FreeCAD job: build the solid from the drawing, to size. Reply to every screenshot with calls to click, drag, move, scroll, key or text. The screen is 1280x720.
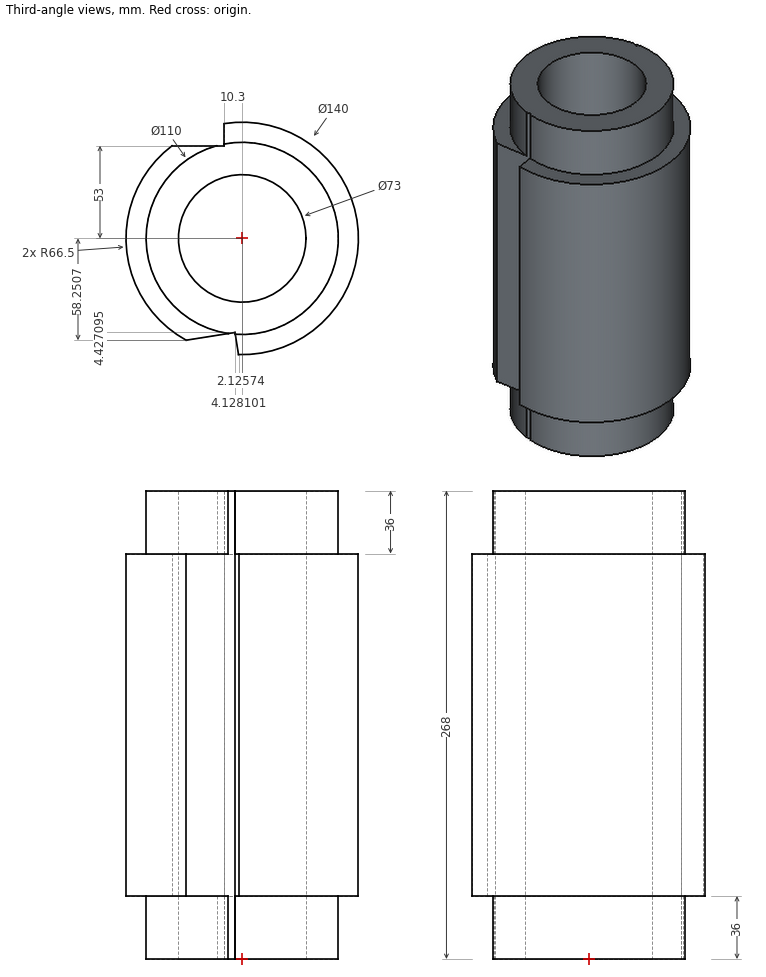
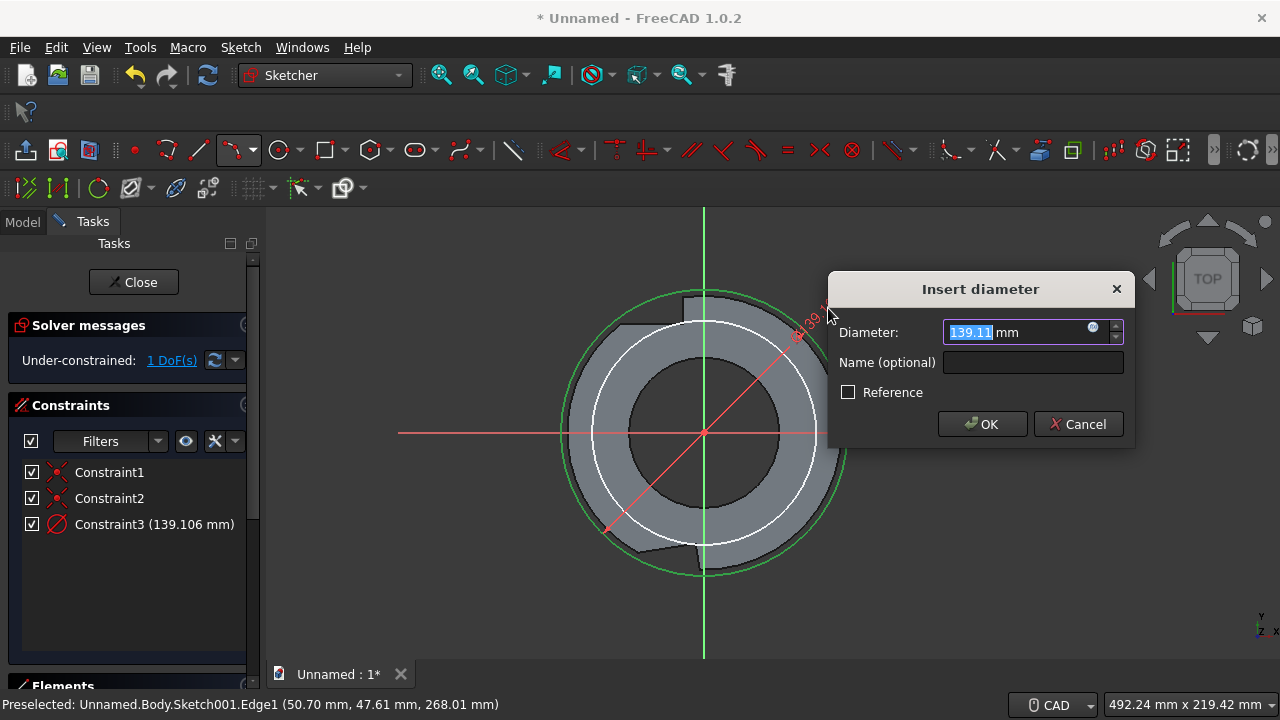
text(140)
key(Return)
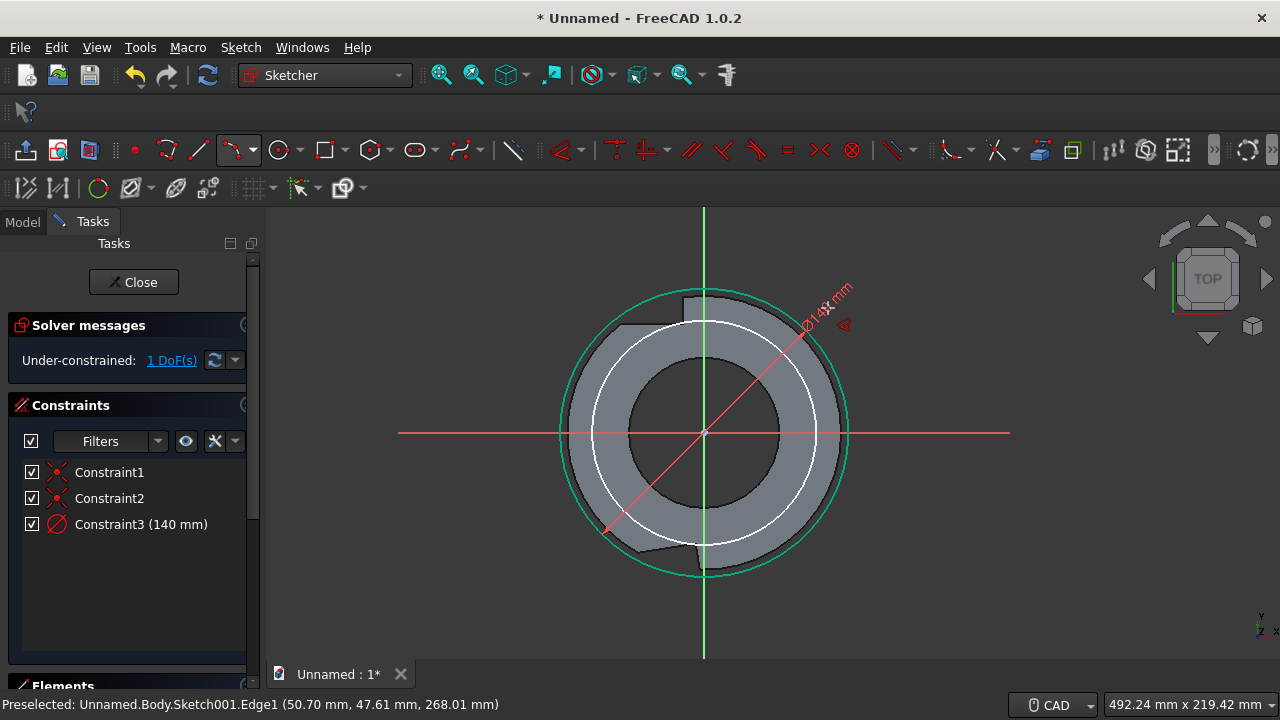
click(783, 353)
click(864, 385)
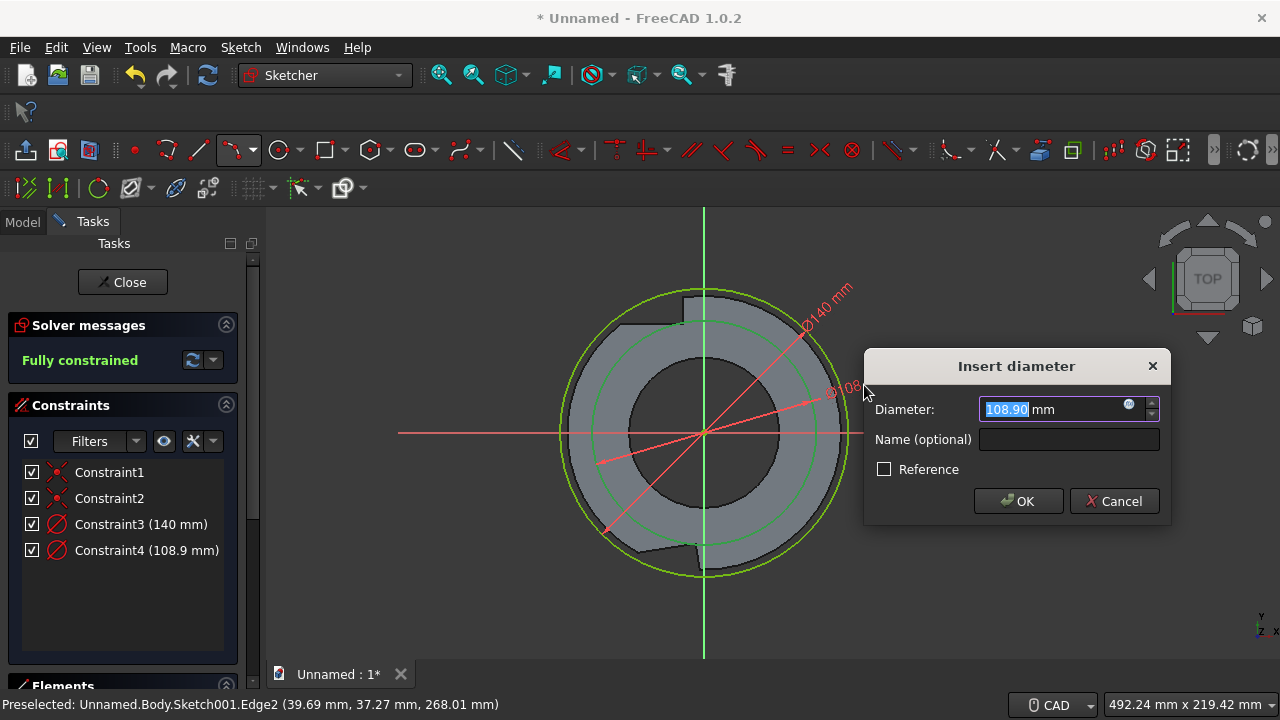
text(110)
key(Return)
key(Escape)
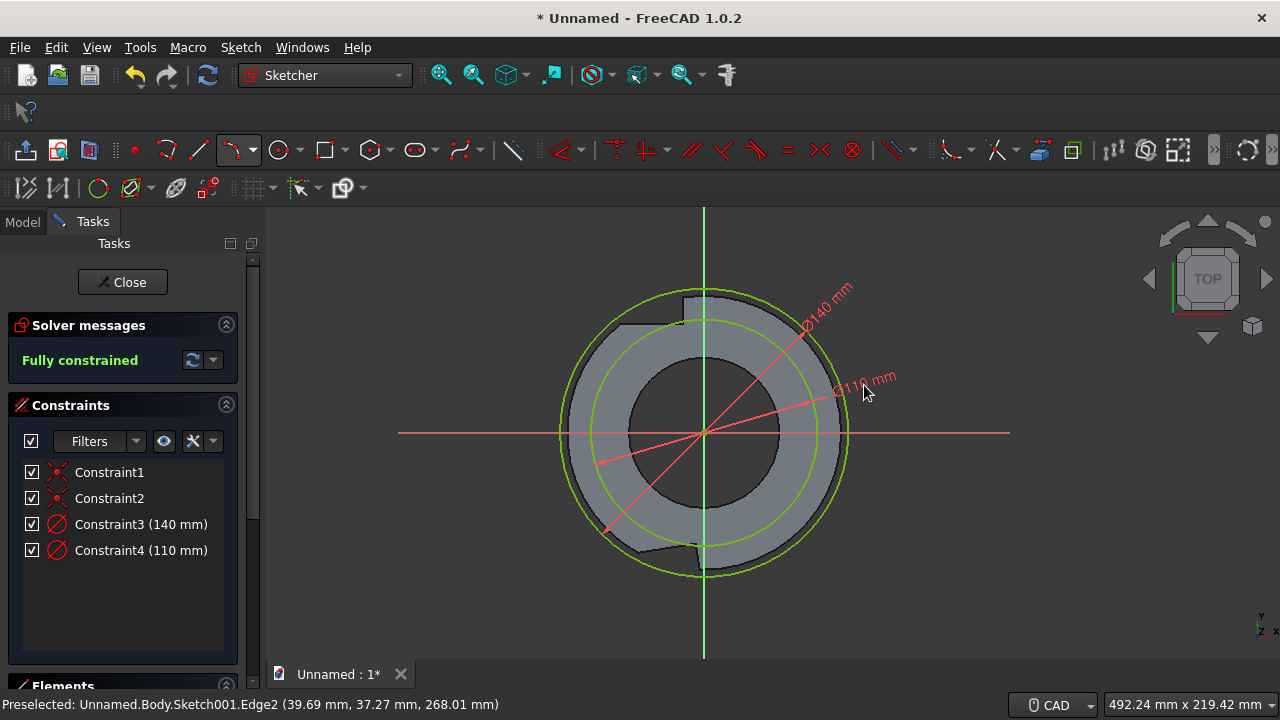
click(123, 282)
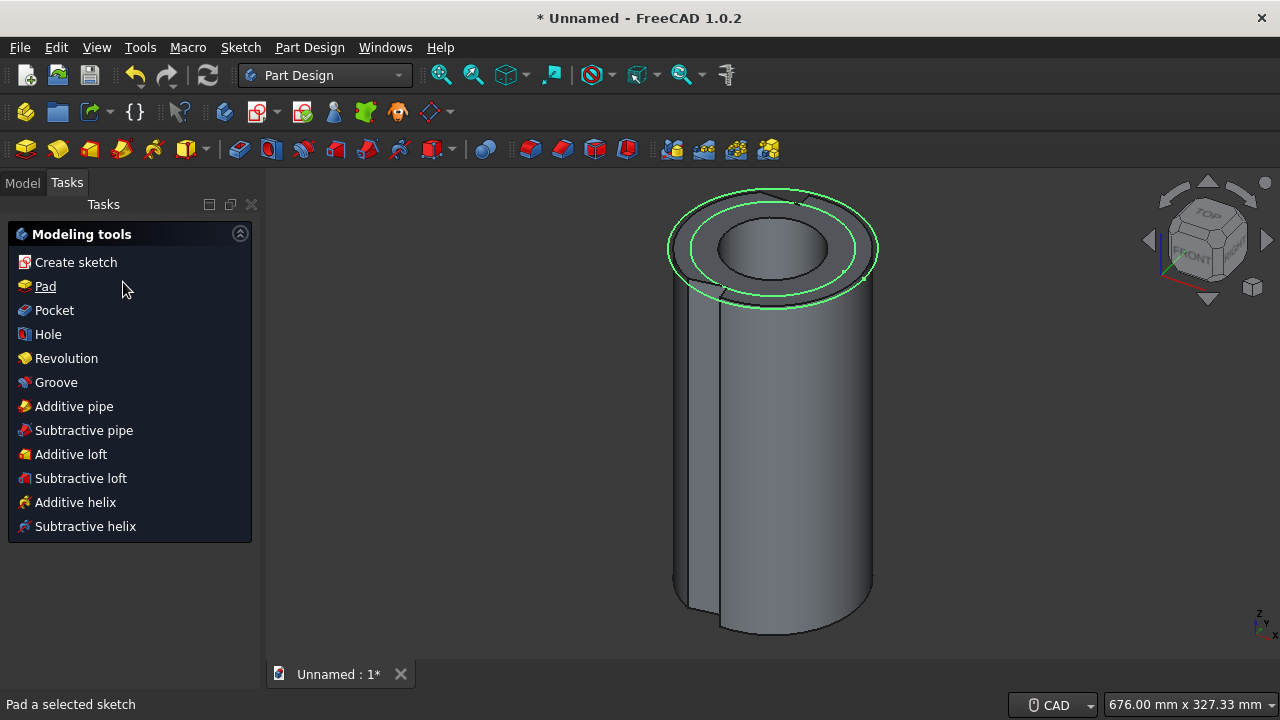
click(240, 150)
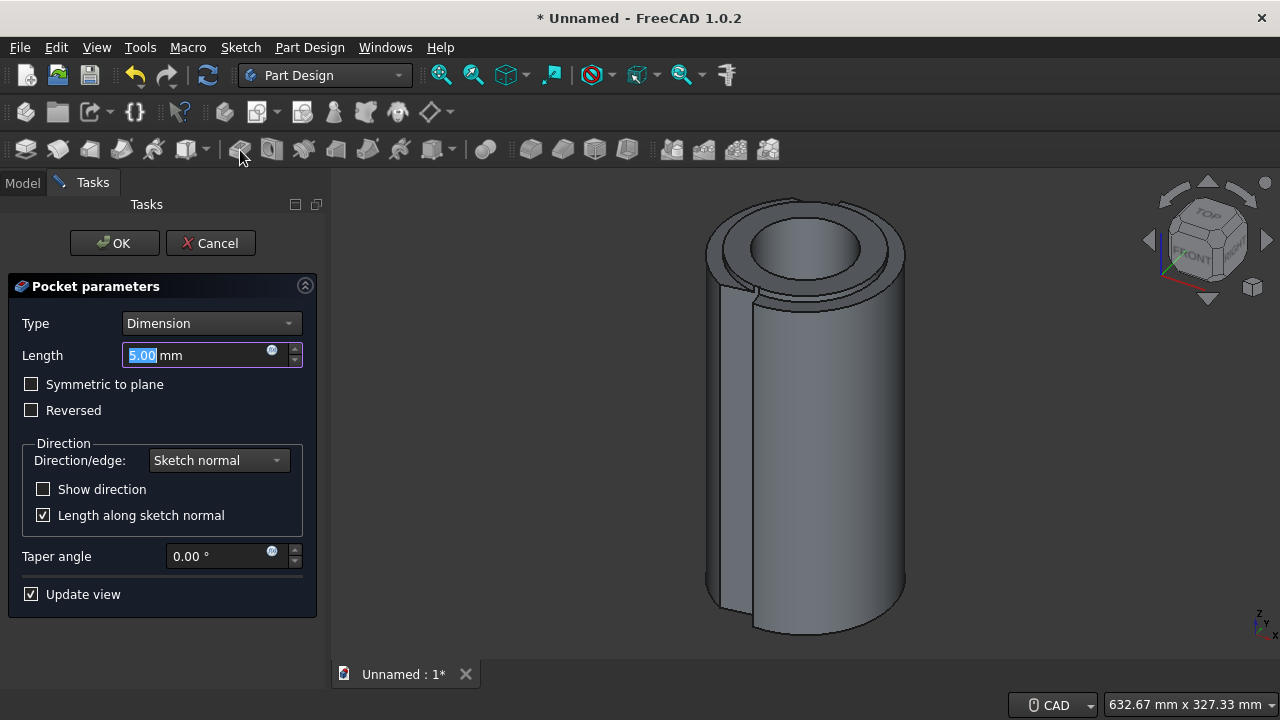
text(36)
key(Tab)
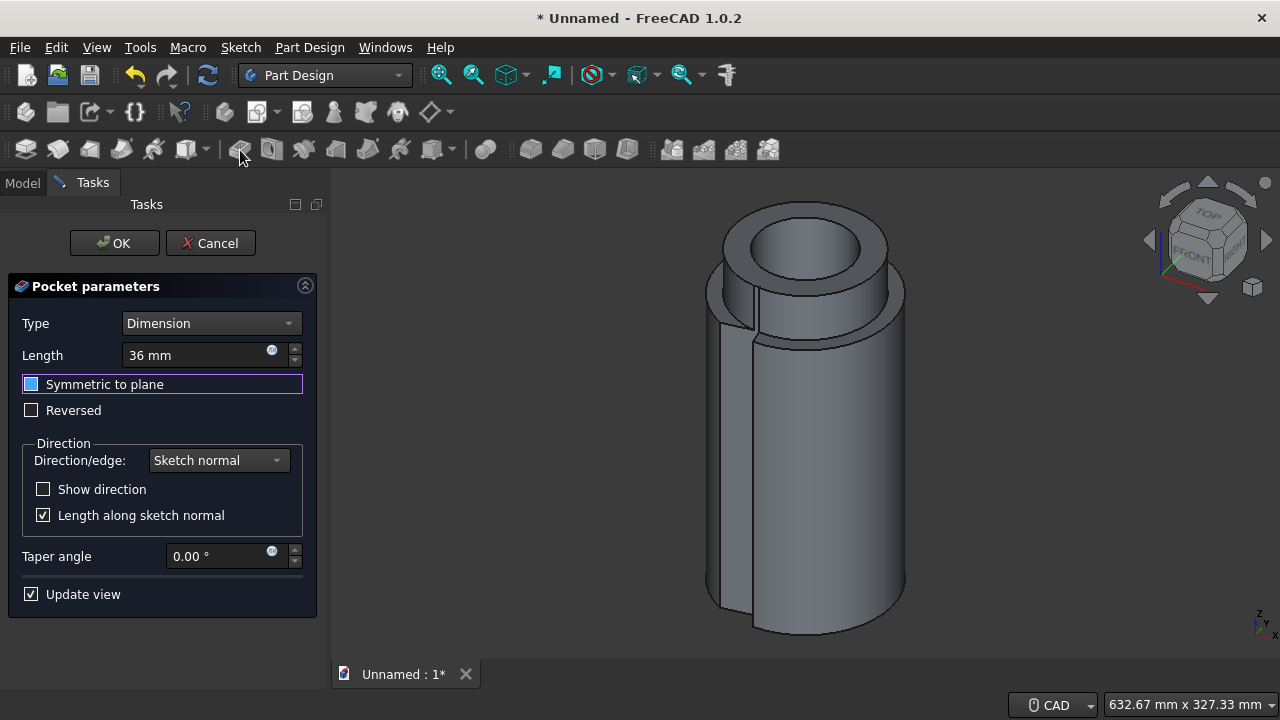
click(115, 243)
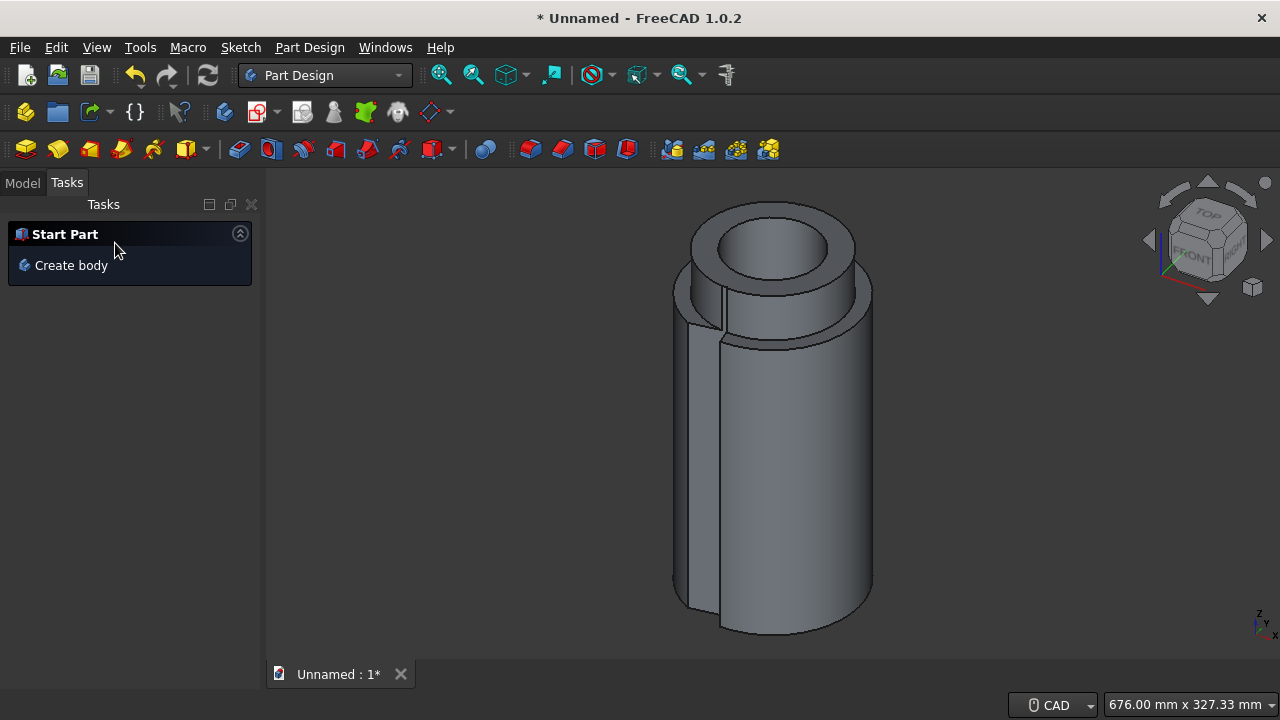
click(23, 182)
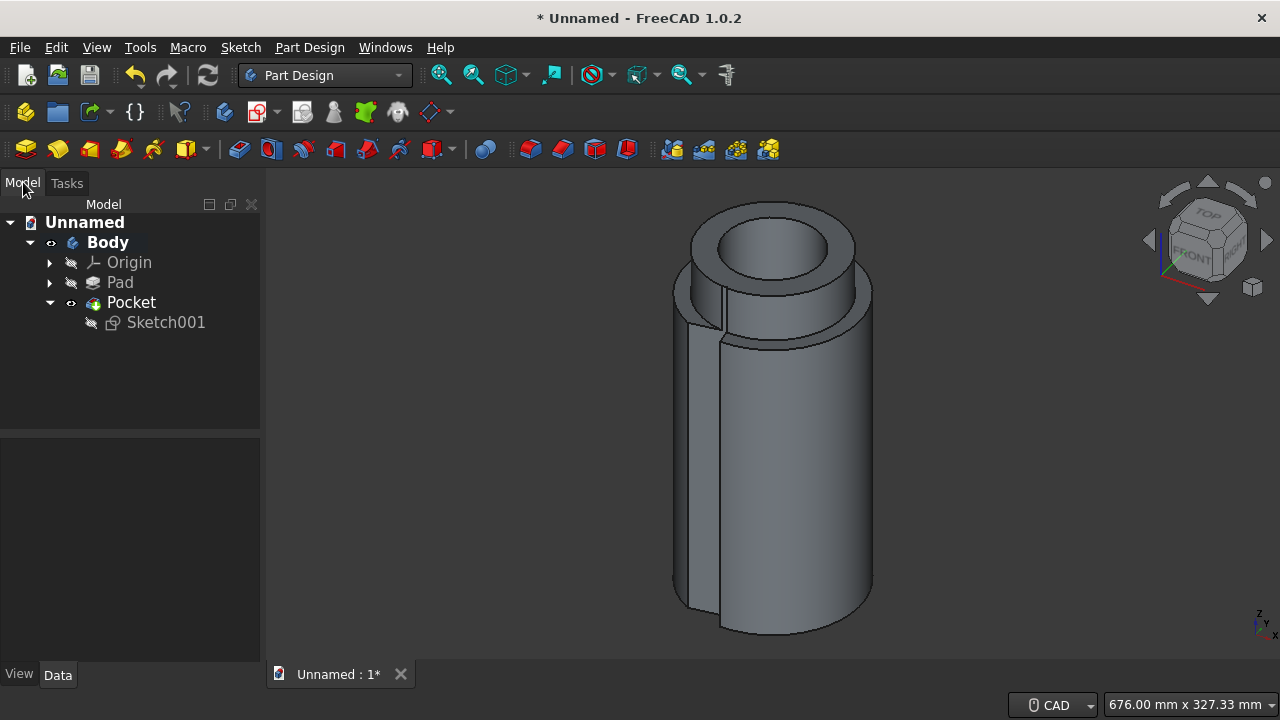
click(50, 263)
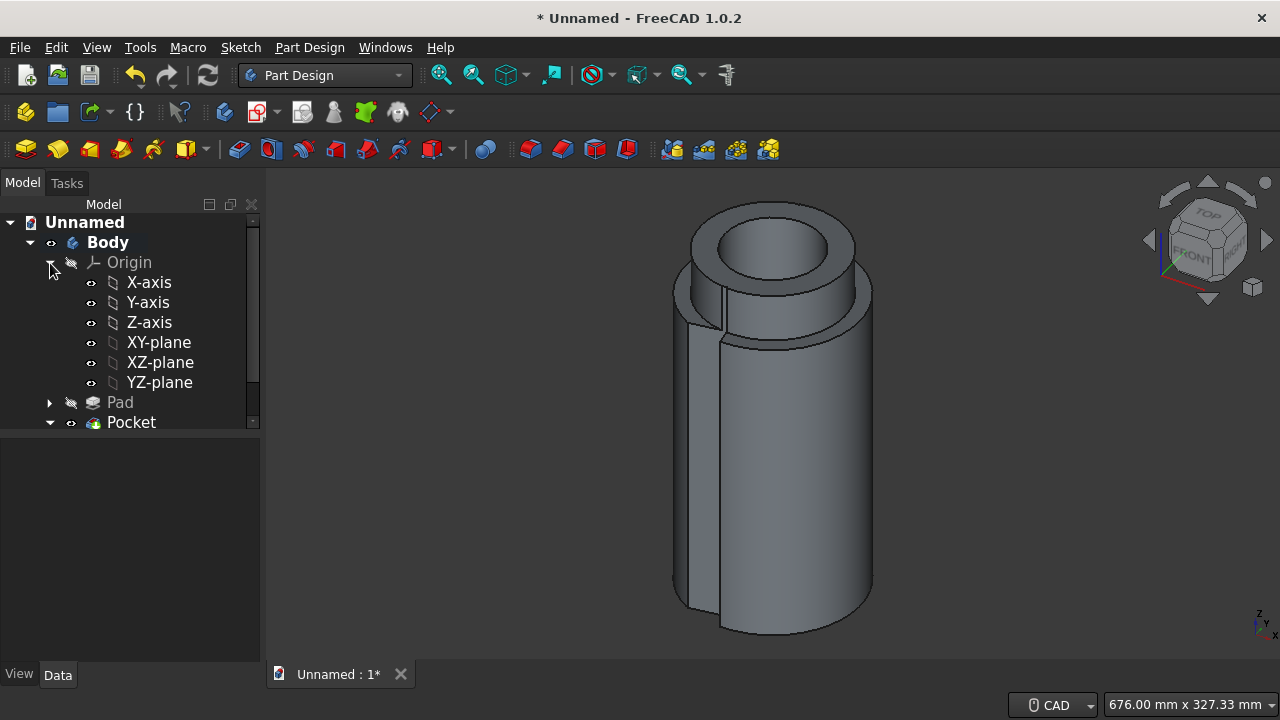
click(136, 343)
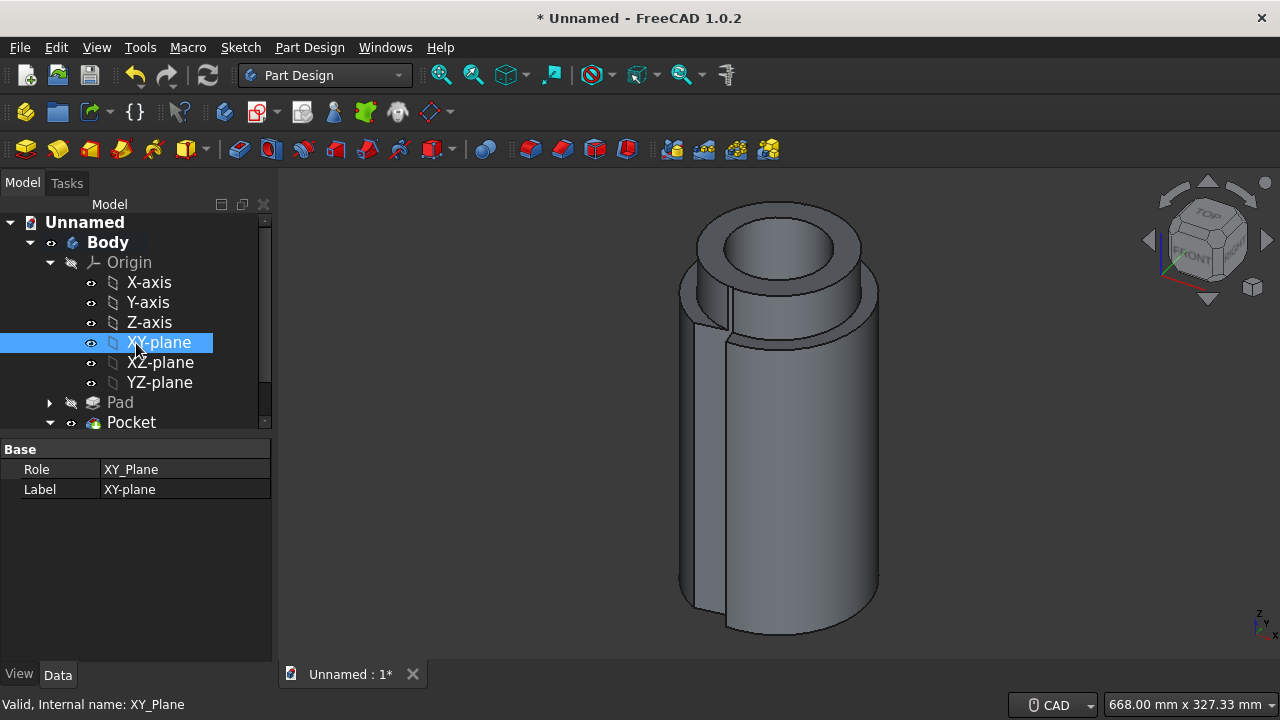
click(430, 112)